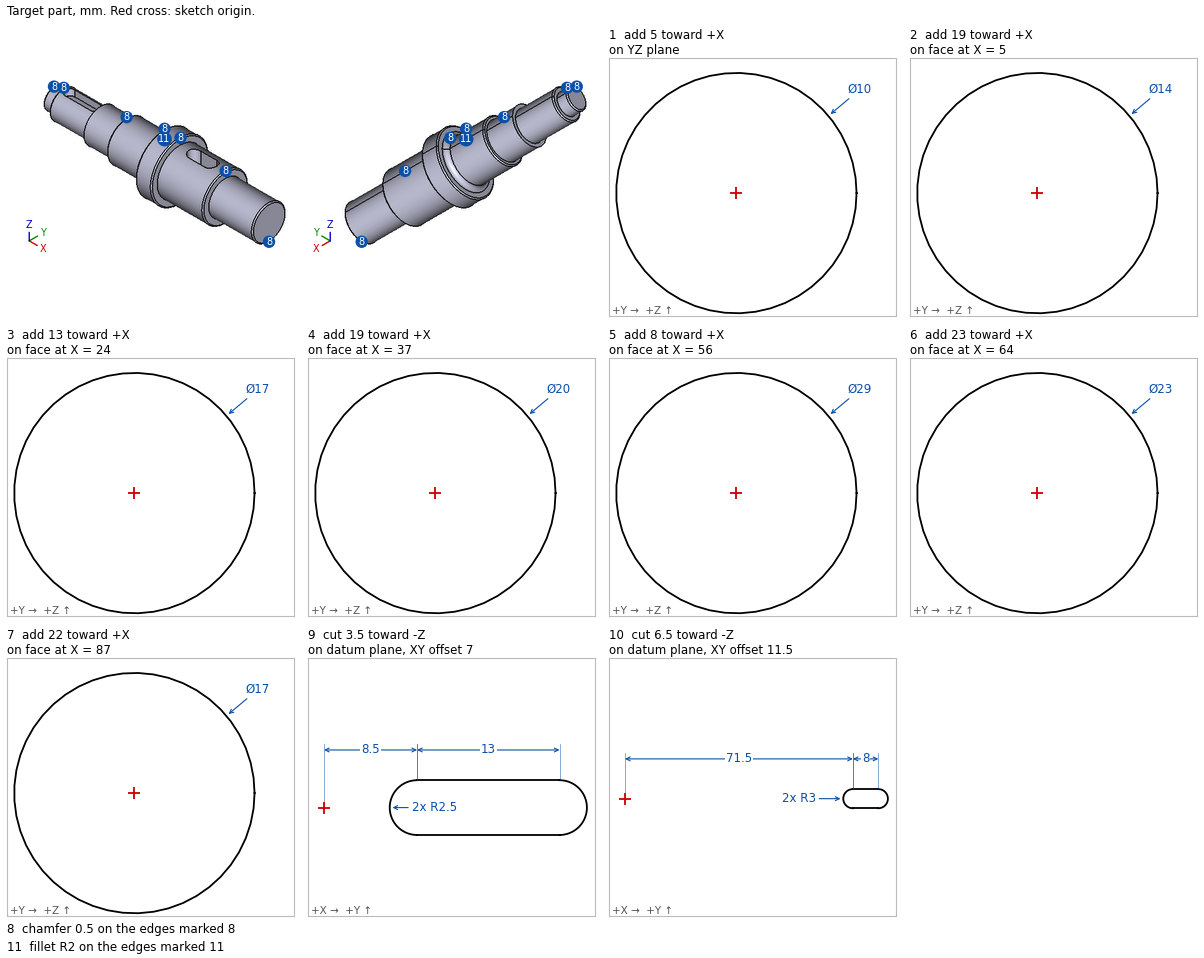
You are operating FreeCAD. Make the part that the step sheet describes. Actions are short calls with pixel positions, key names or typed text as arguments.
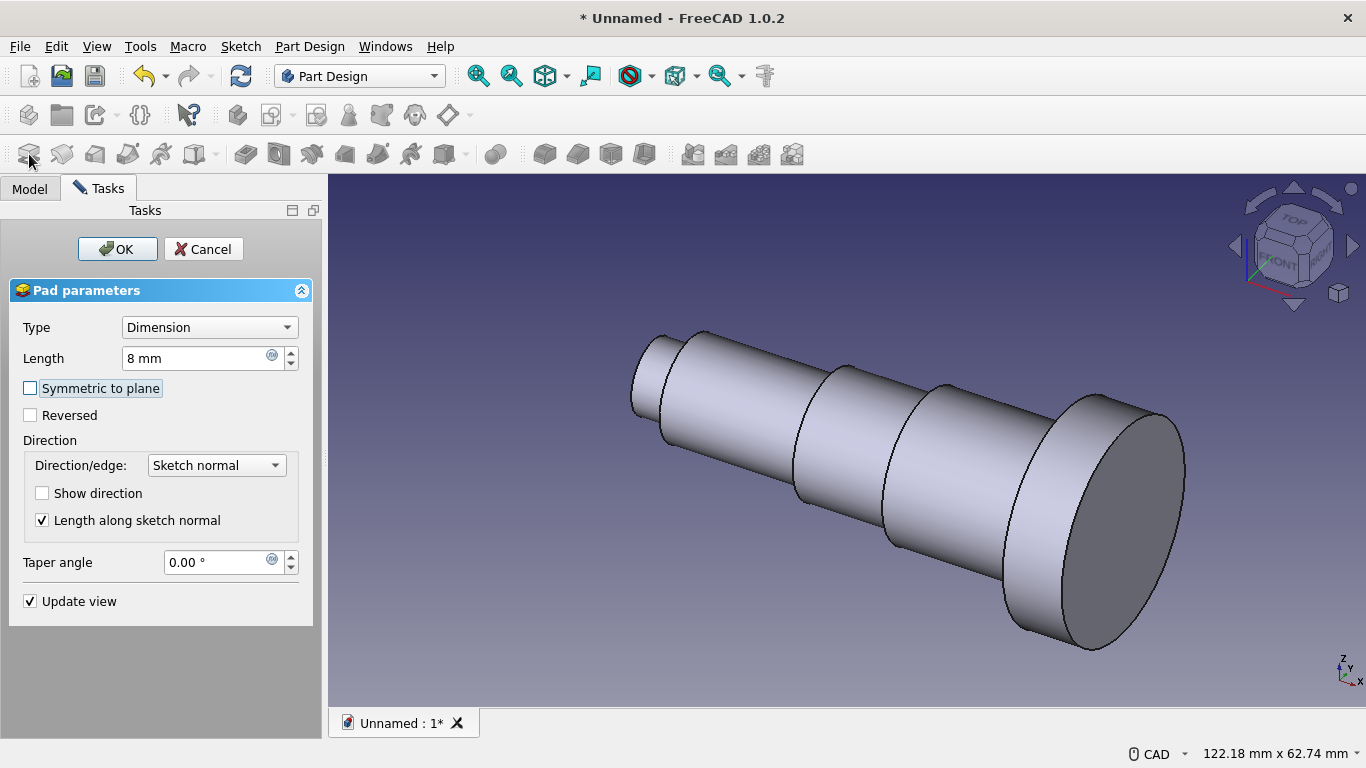
click(118, 249)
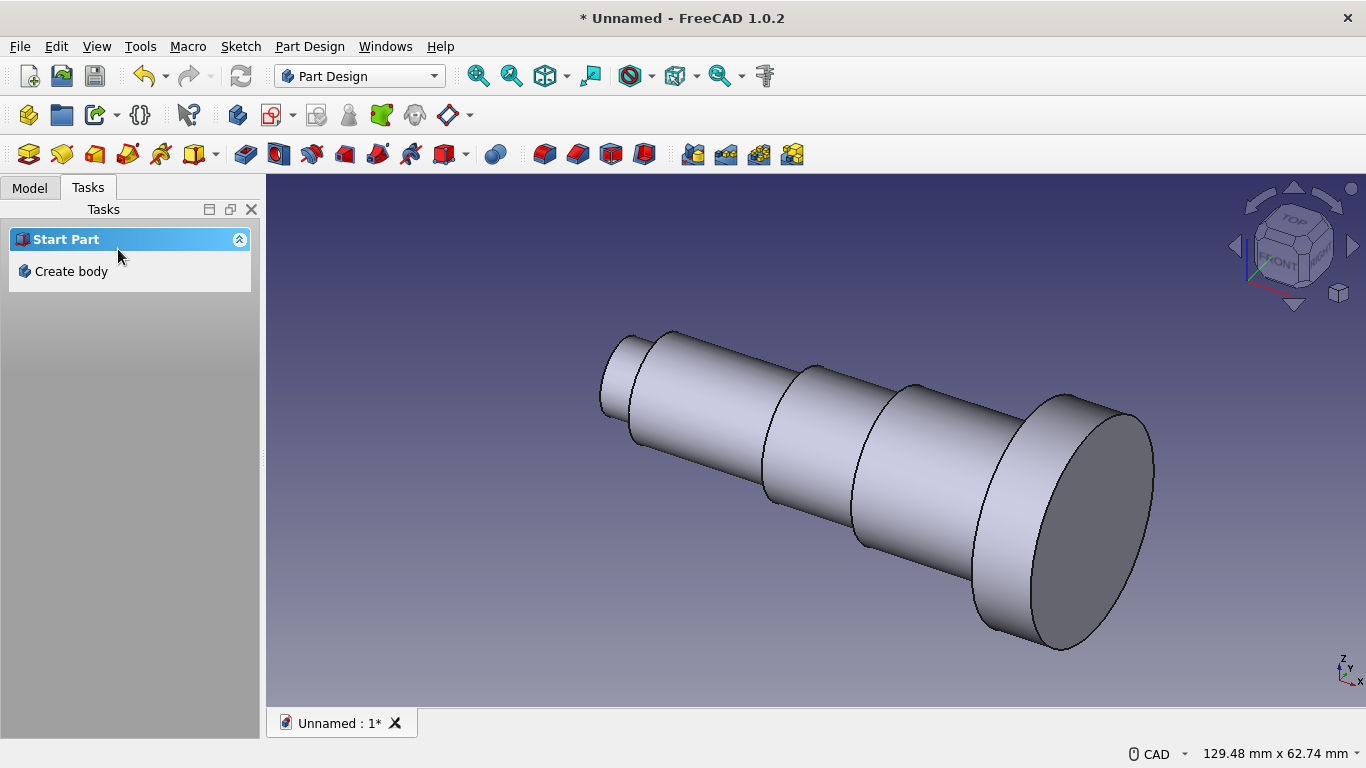
click(1092, 531)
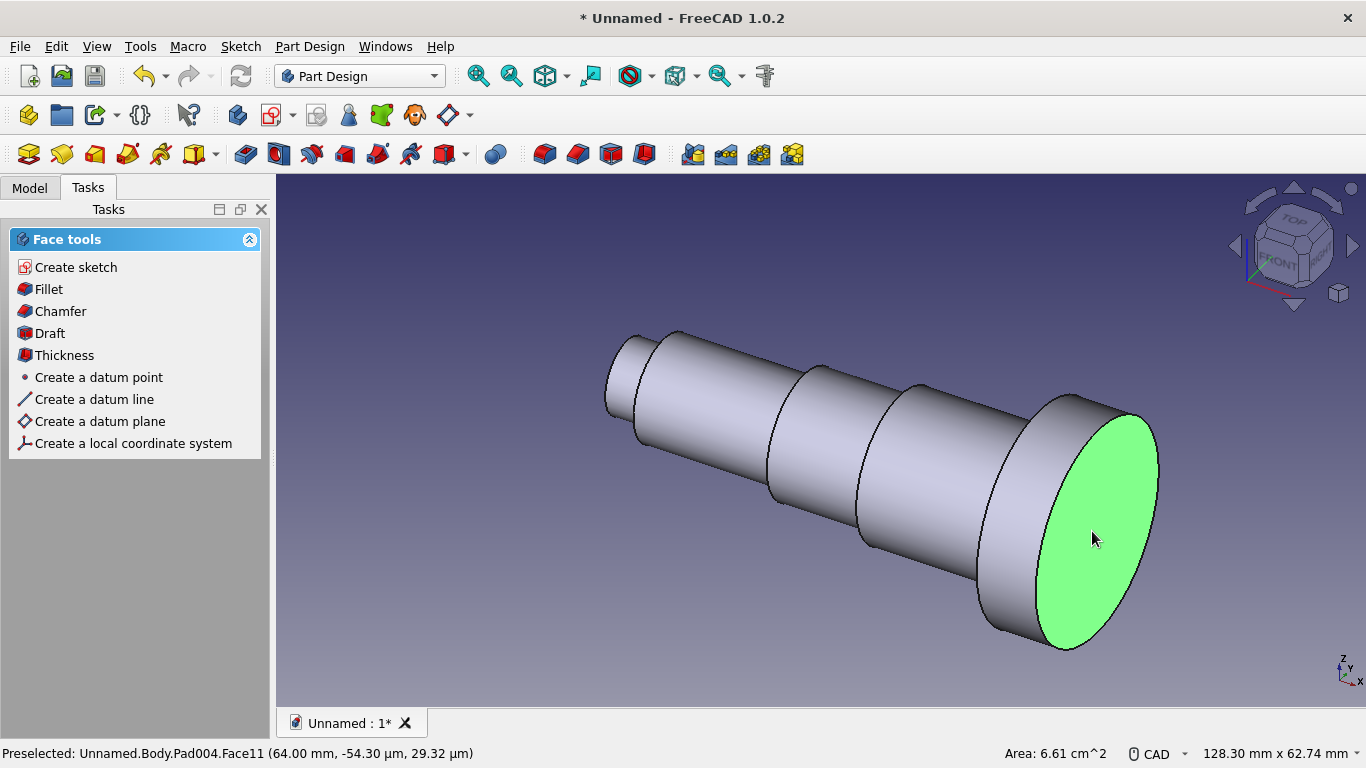
click(270, 116)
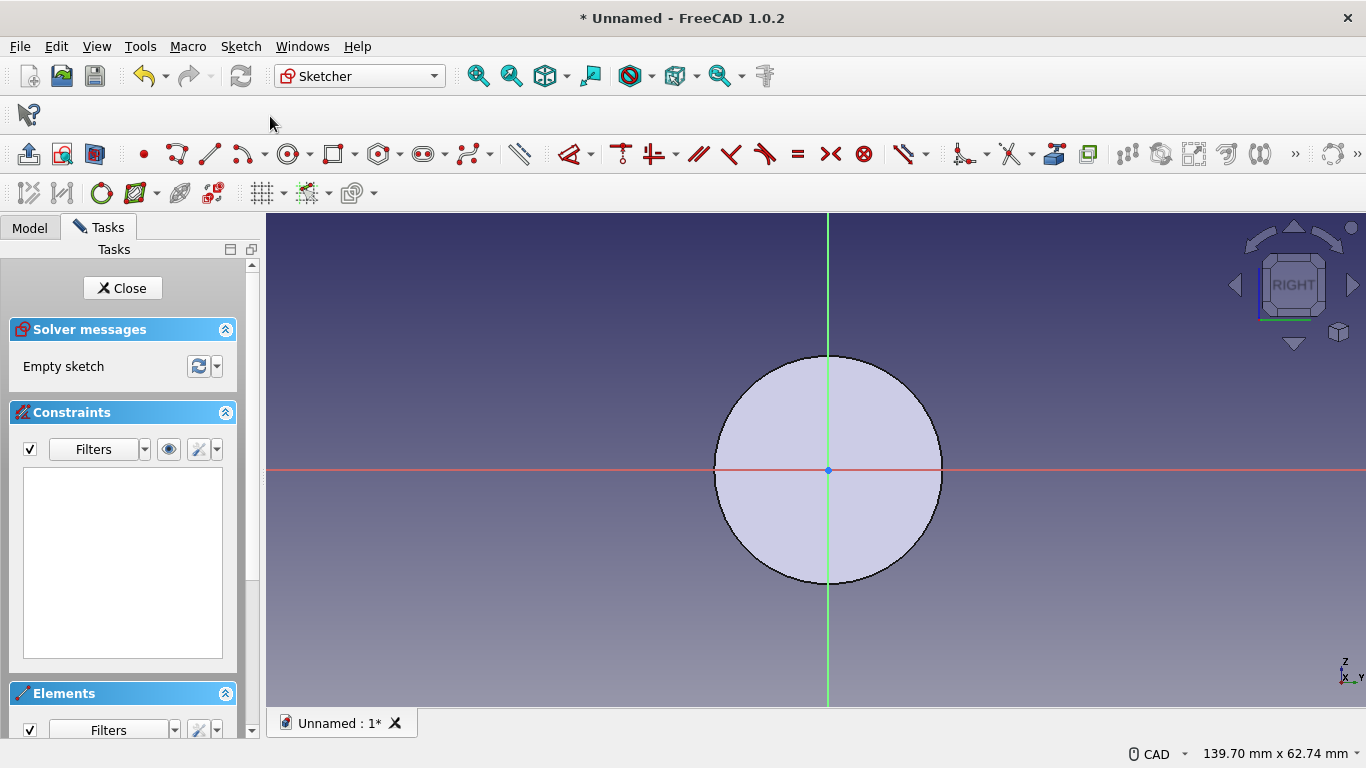
scroll(927, 482, up, 3)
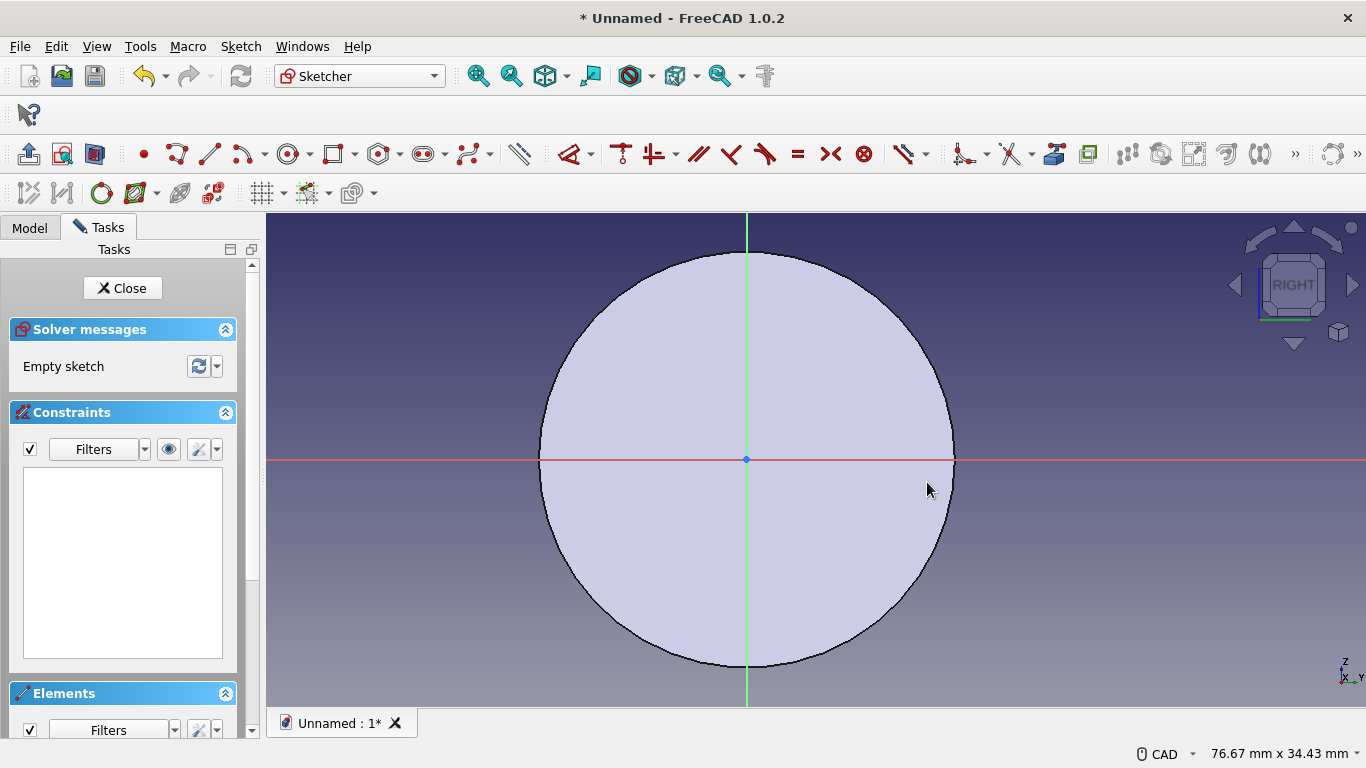
key(g)
key(c)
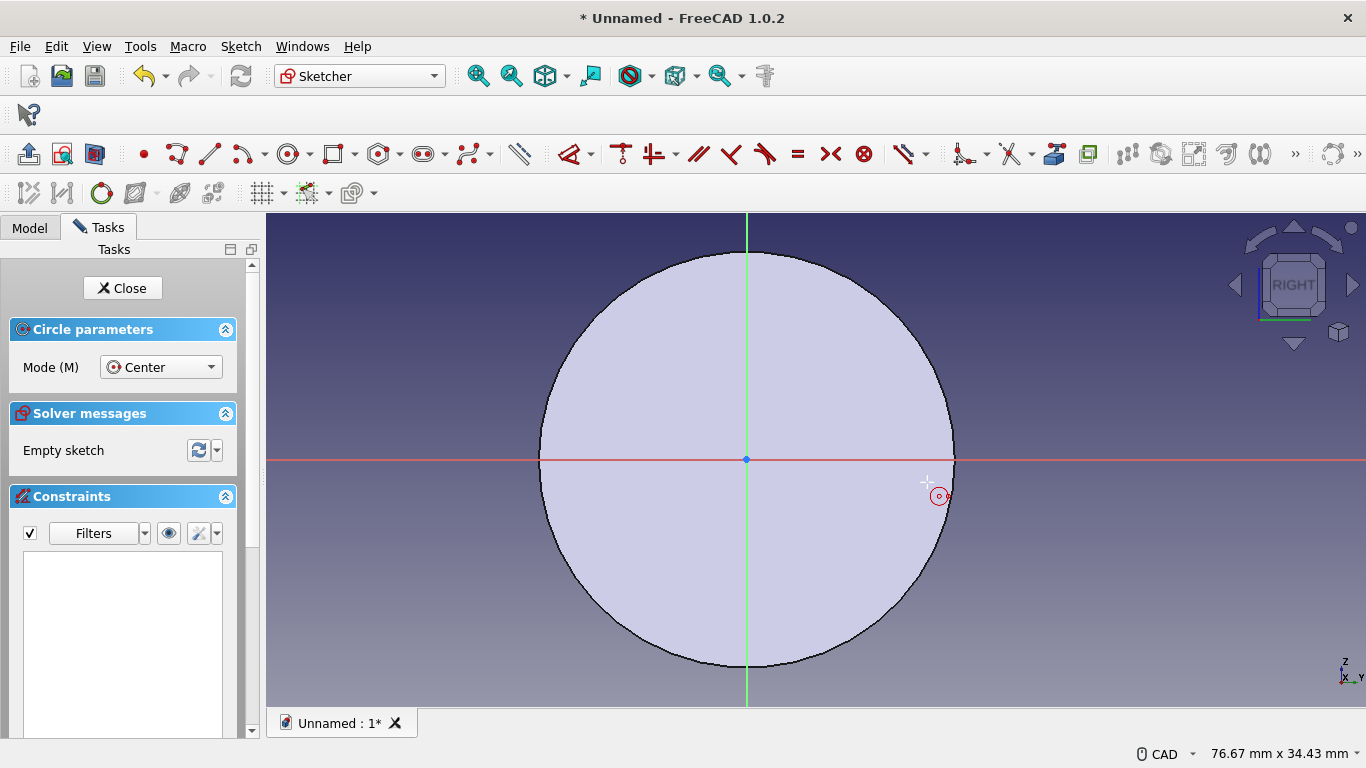
click(747, 460)
move(864, 343)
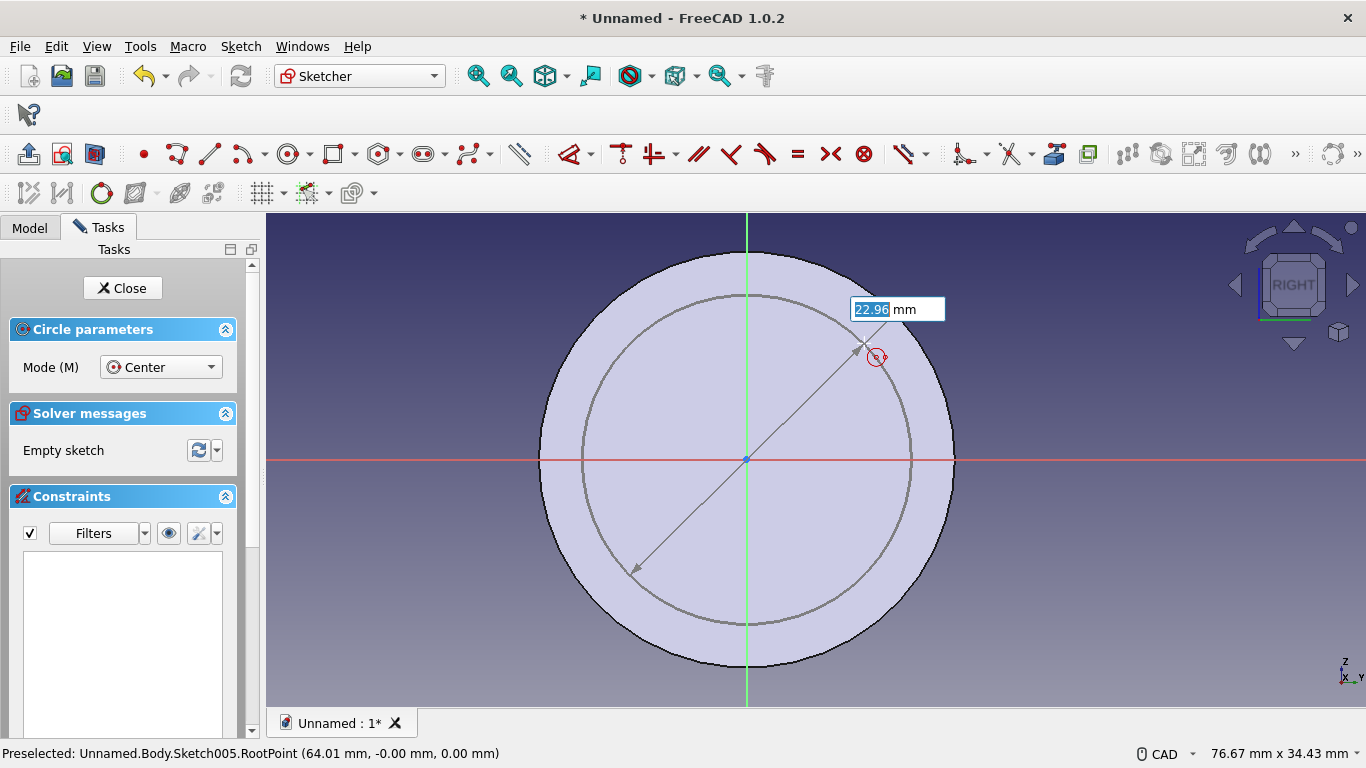
text(23)
key(Return)
key(Escape)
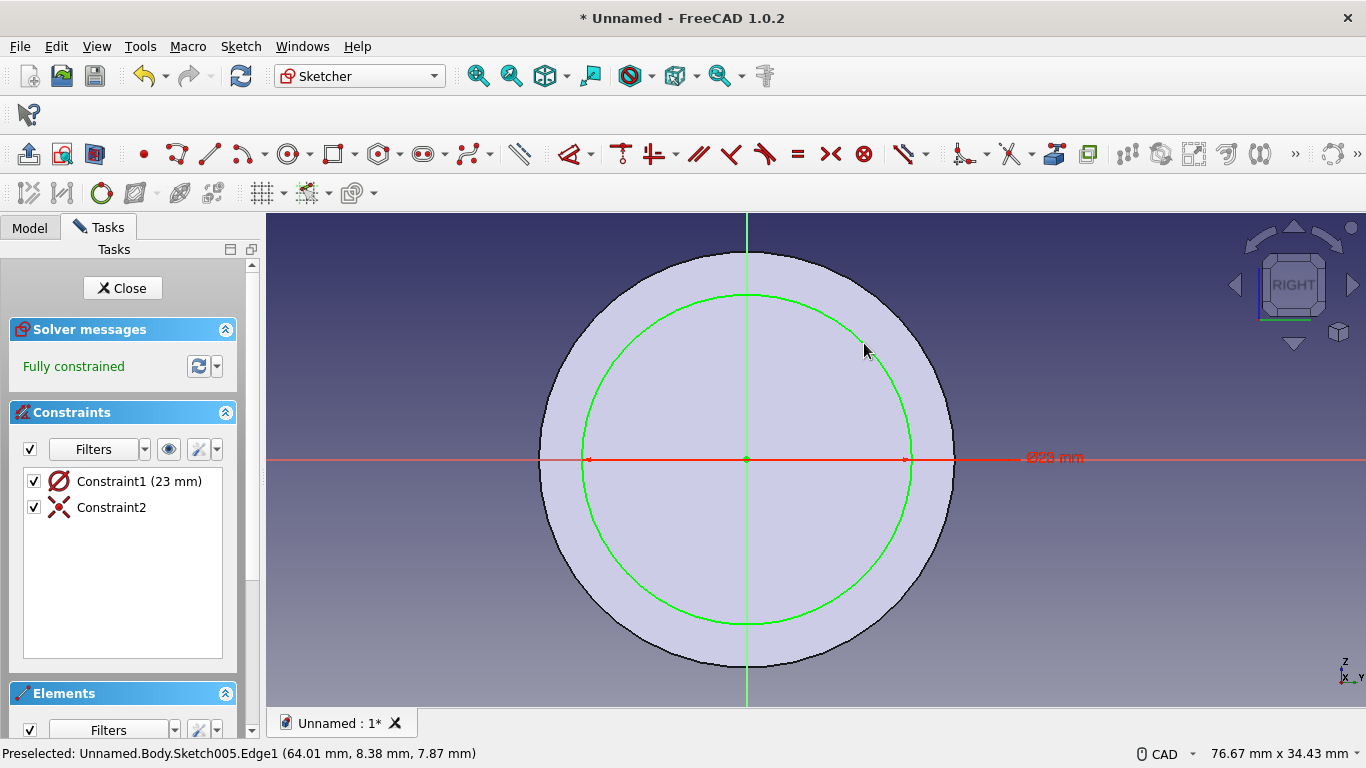
click(123, 288)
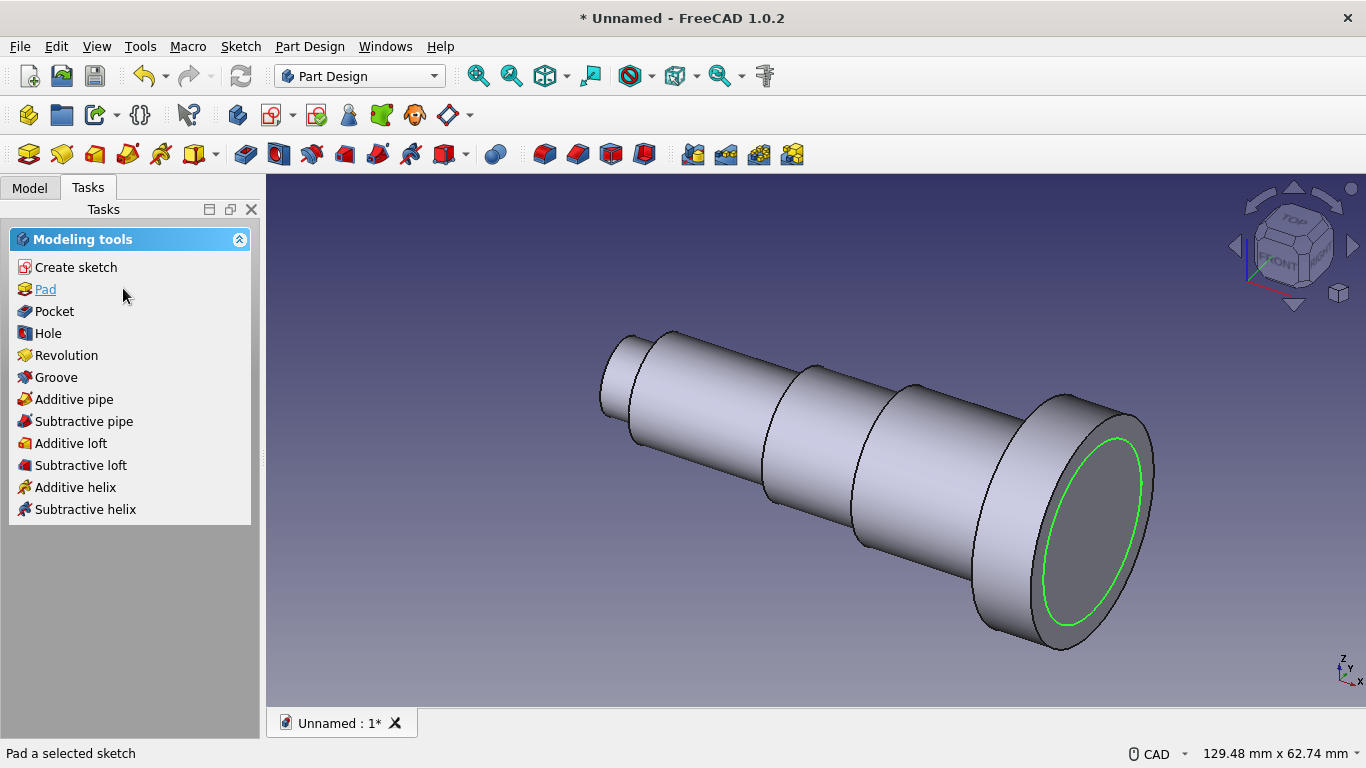
click(29, 154)